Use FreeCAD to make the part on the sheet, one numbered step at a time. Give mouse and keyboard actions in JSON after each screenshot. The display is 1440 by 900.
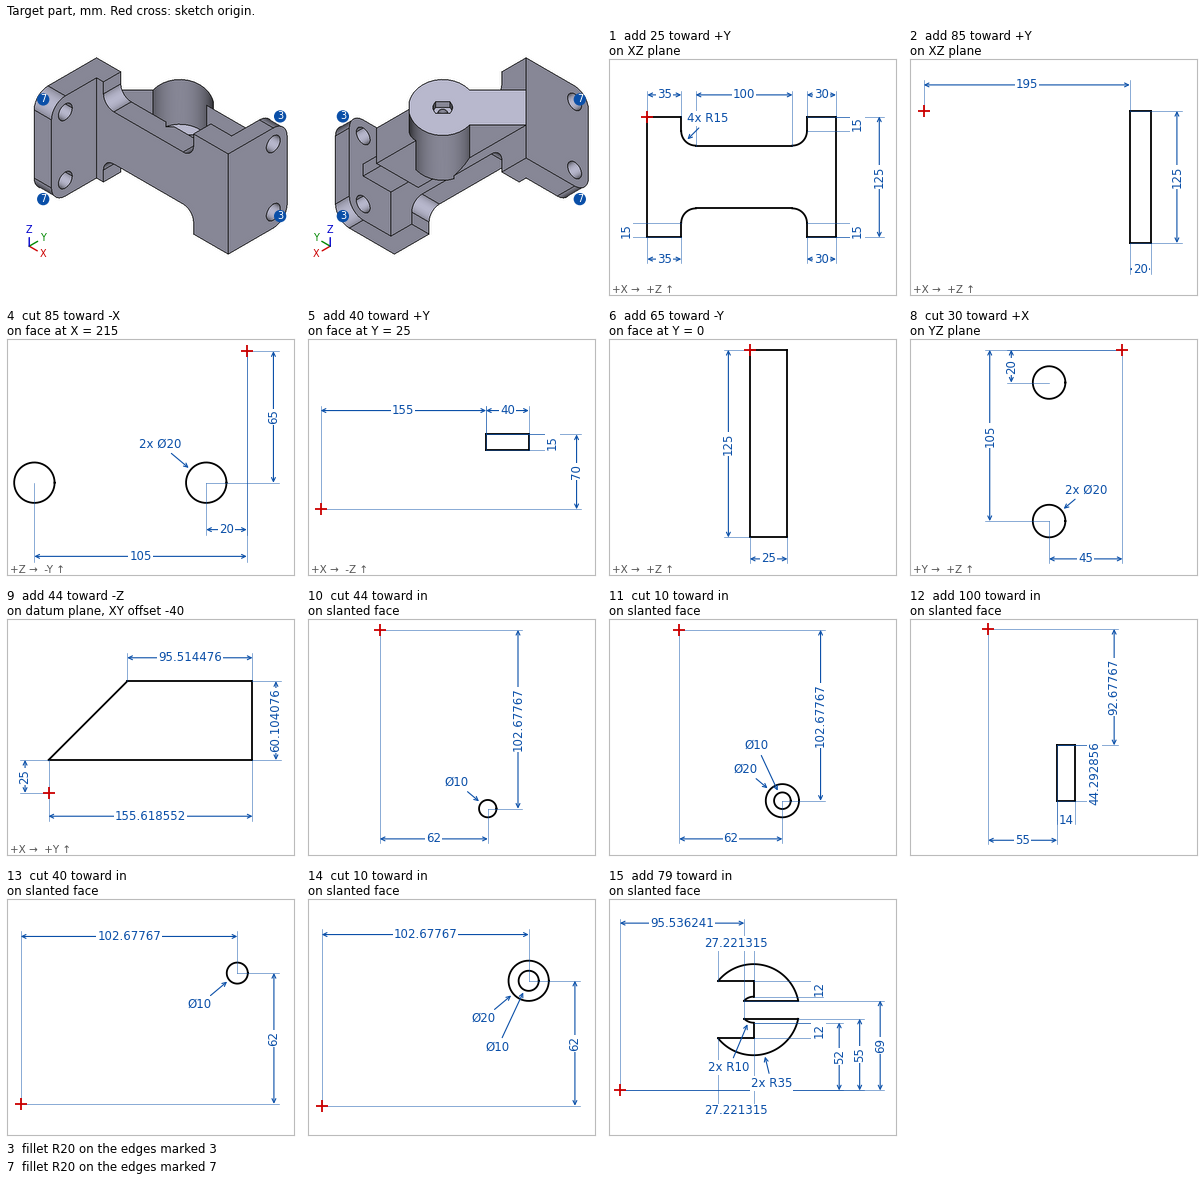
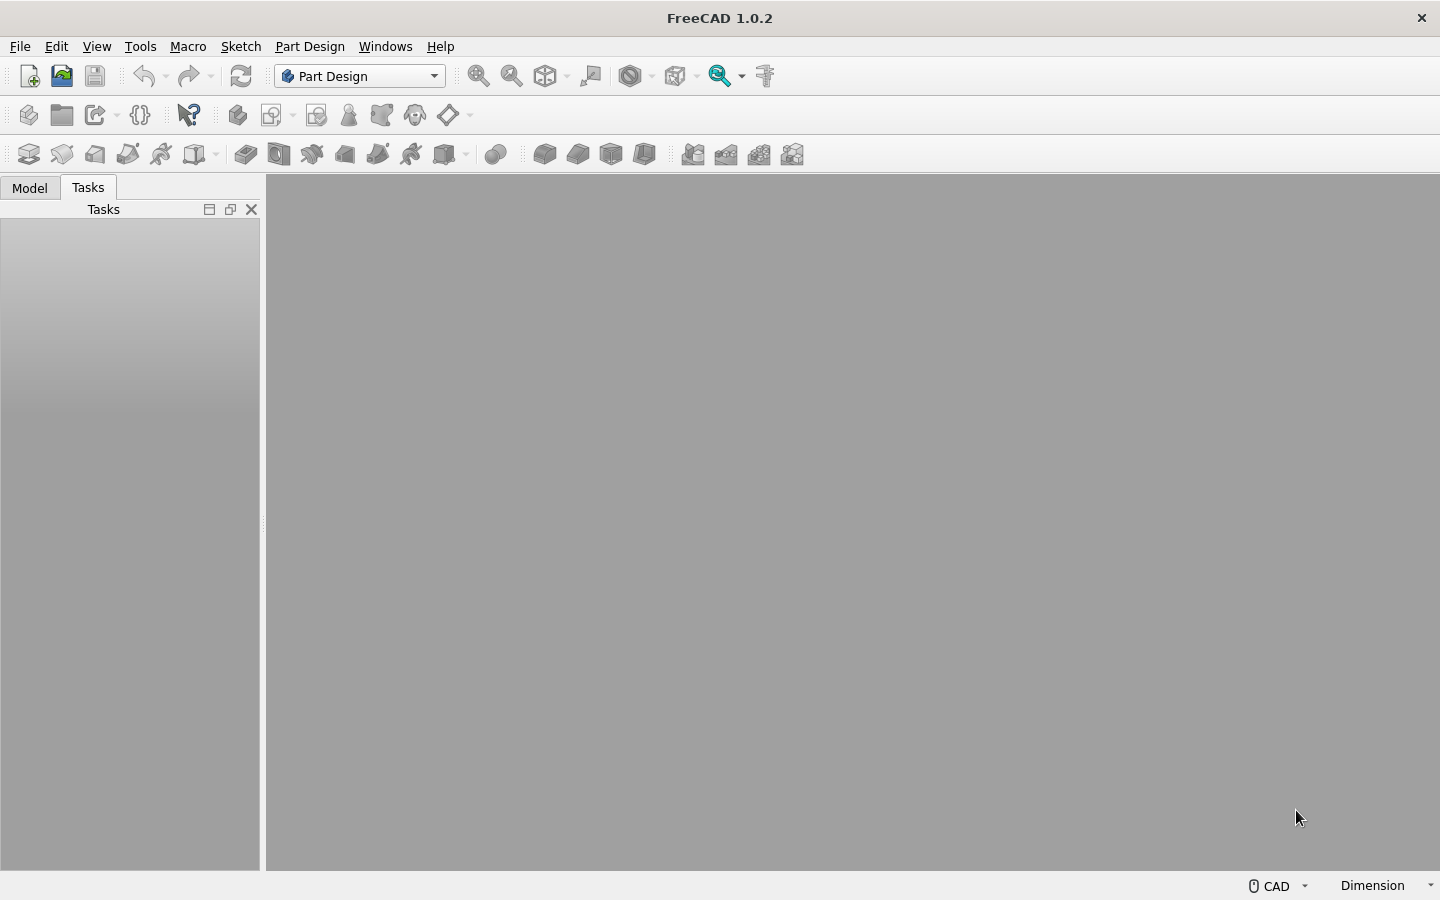
{"action": "left_click", "coordinate": [29, 76]}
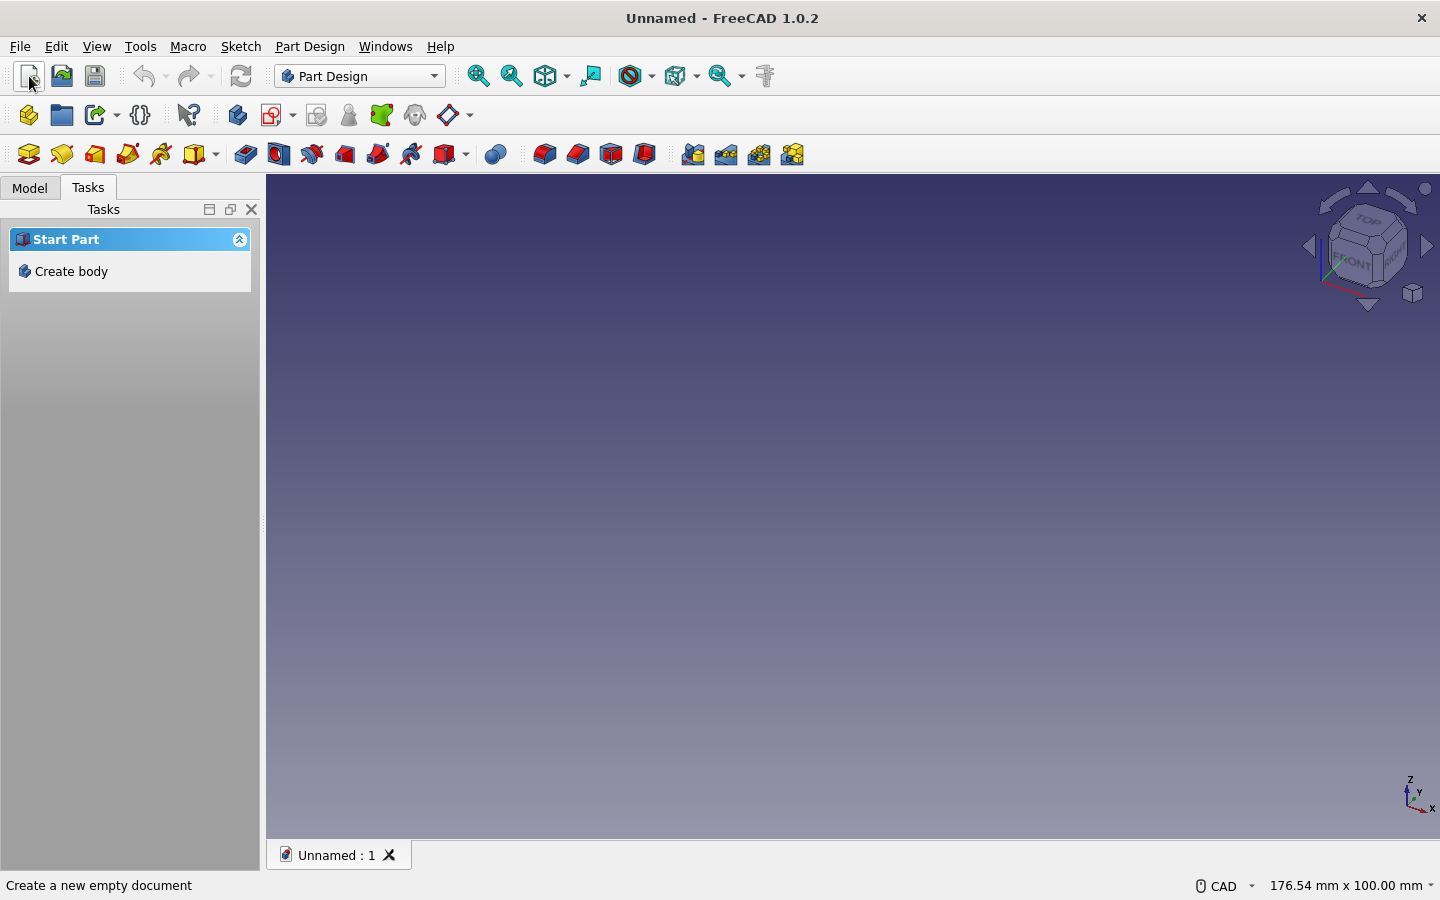
{"action": "left_click", "coordinate": [270, 116]}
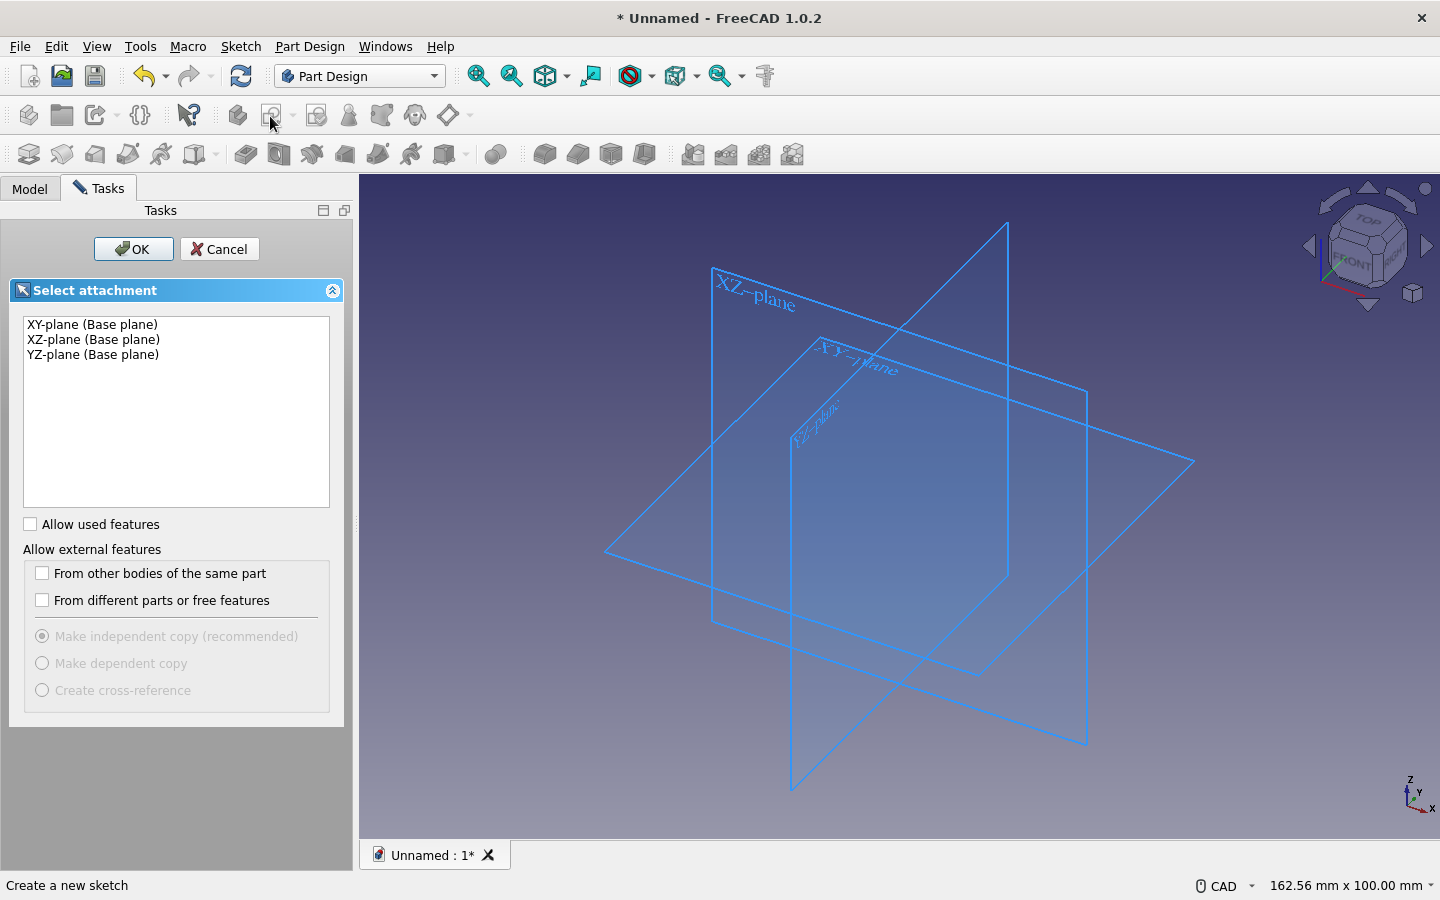
{"action": "left_click", "coordinate": [84, 340]}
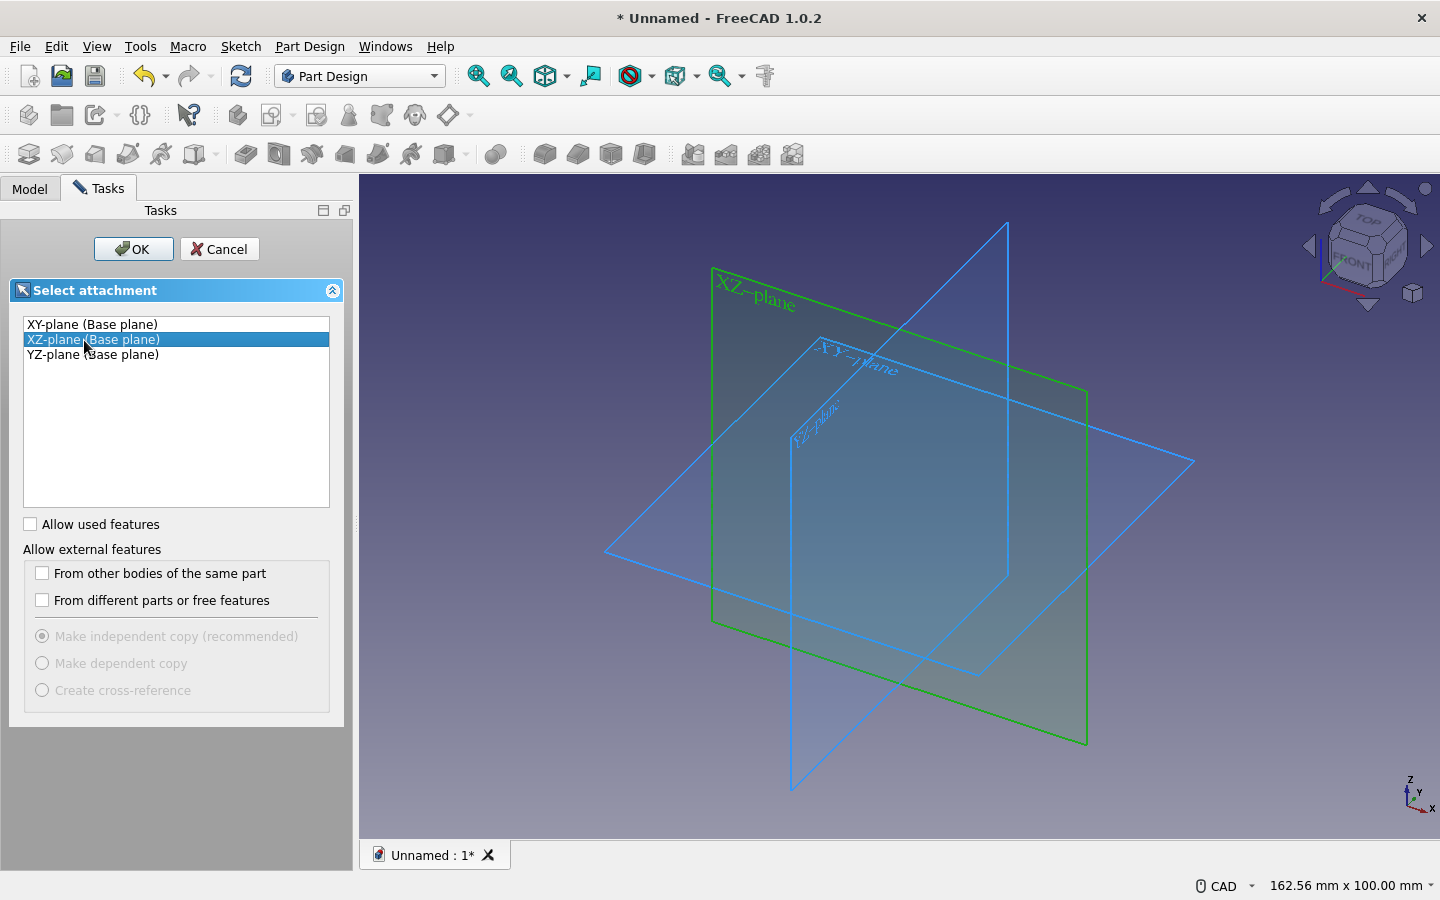
{"action": "left_click", "coordinate": [134, 249]}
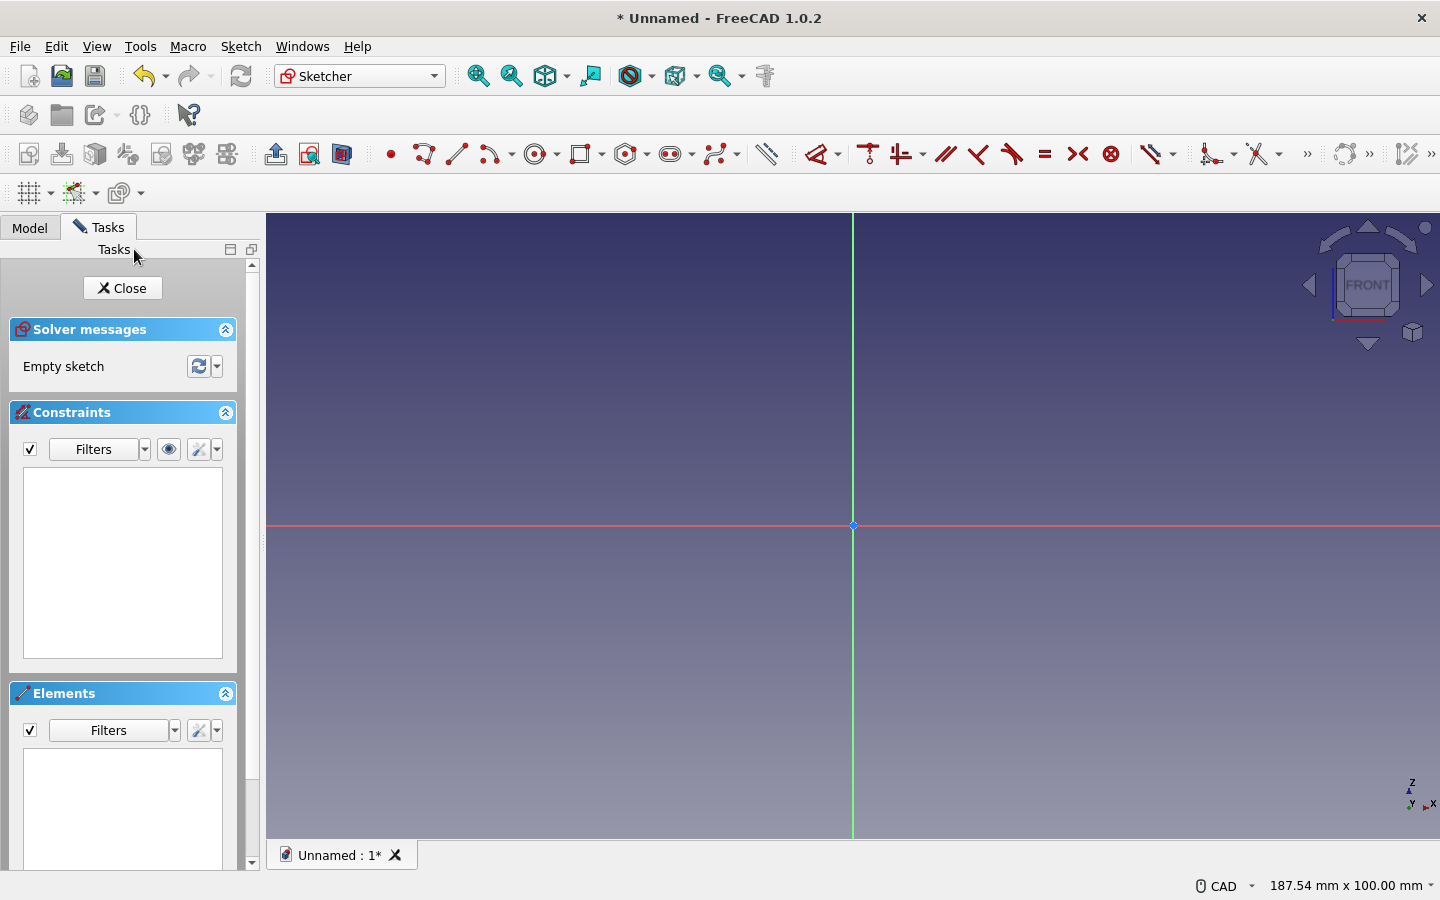
{"action": "scroll", "coordinate": [294, 241], "scroll_direction": "down", "scroll_amount": 4}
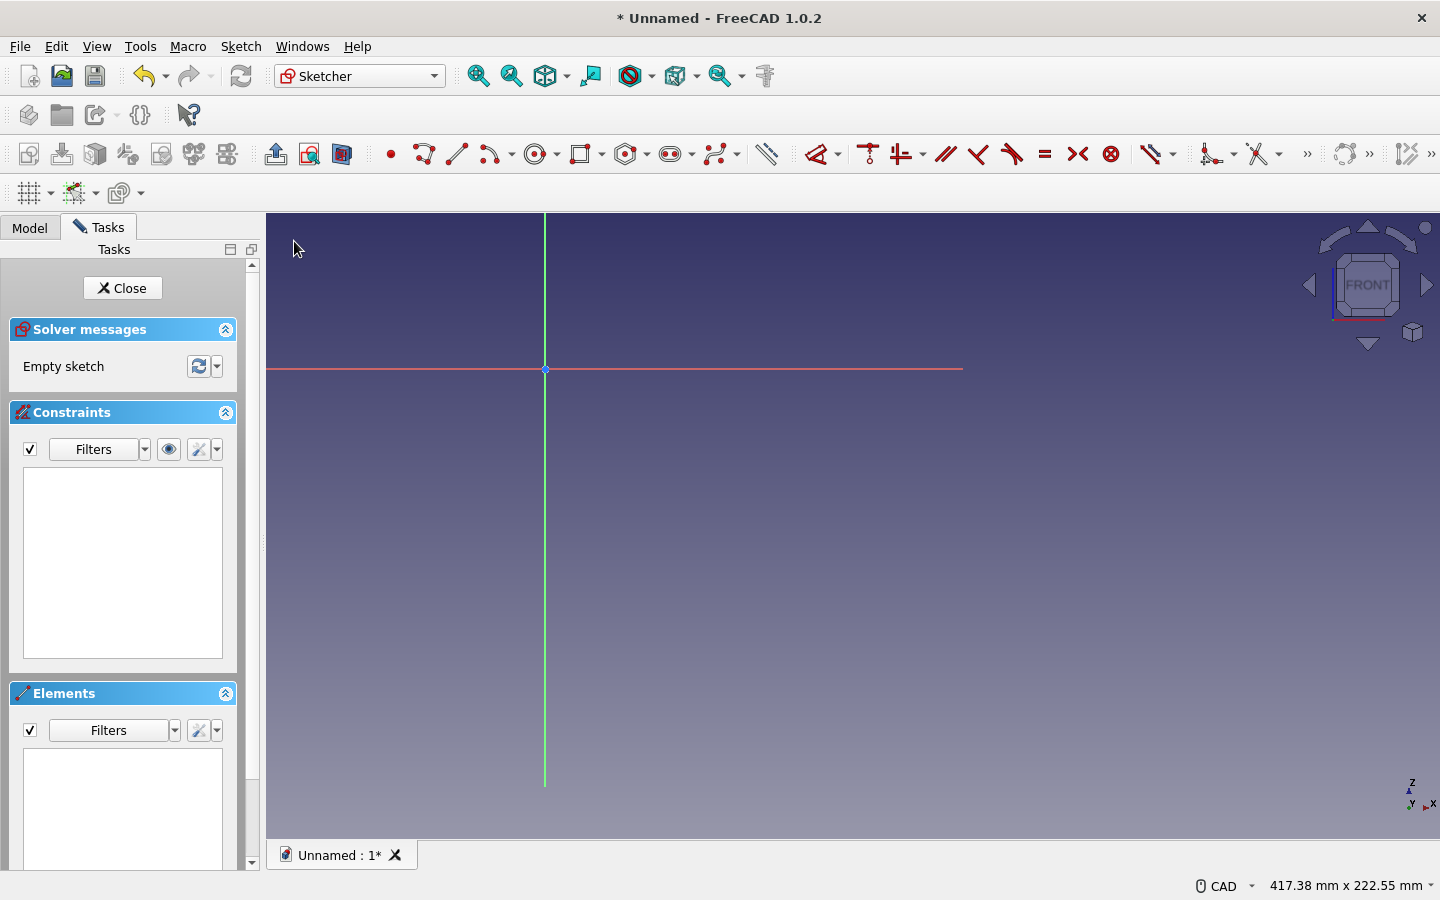
{"action": "left_click", "coordinate": [457, 154]}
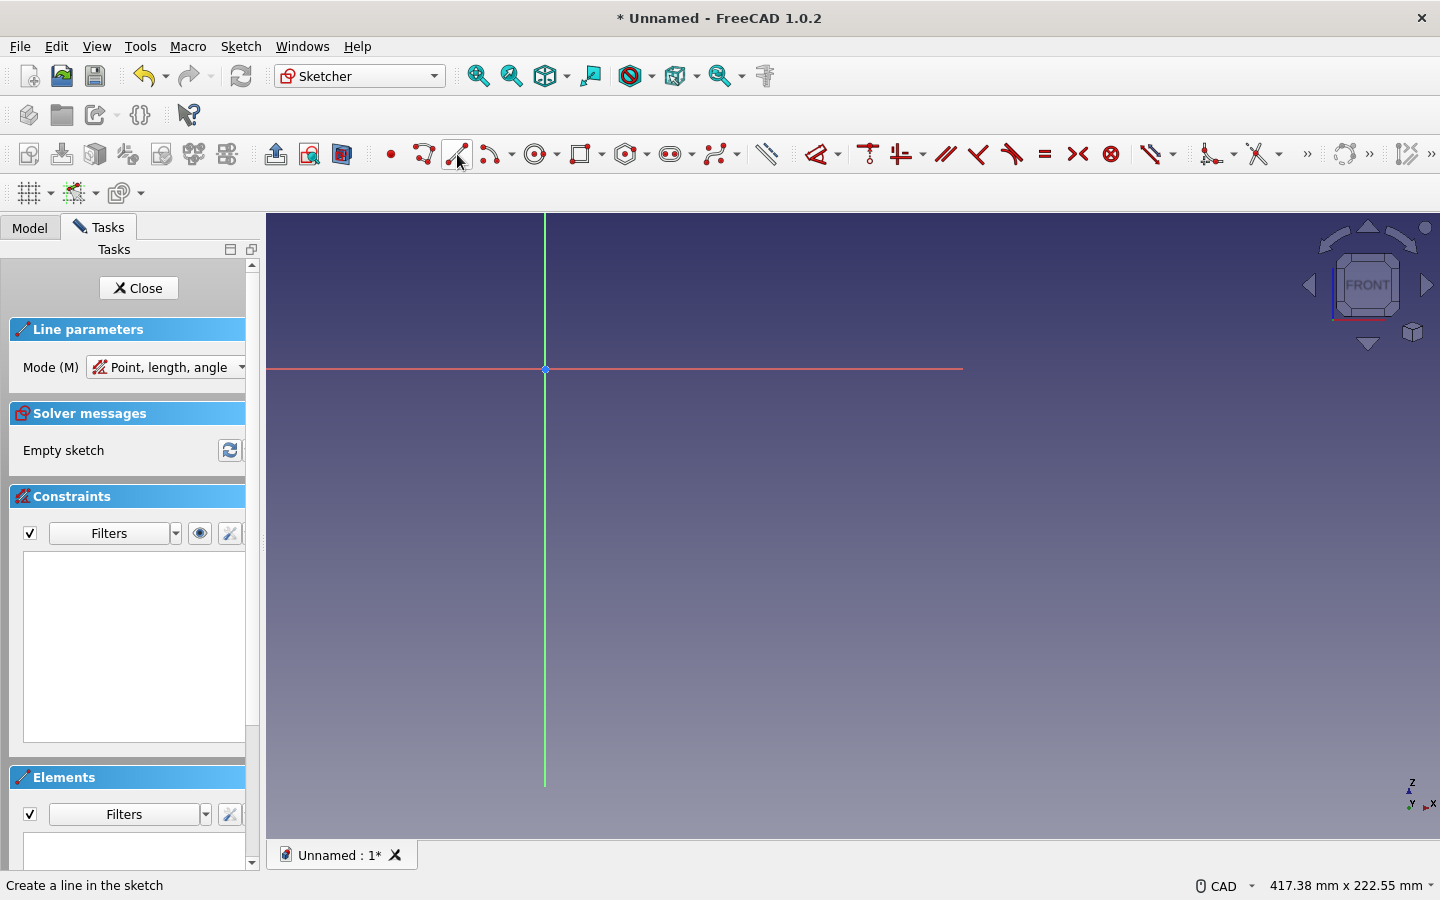
{"action": "left_click", "coordinate": [686, 453]}
{"action": "left_click", "coordinate": [967, 453]}